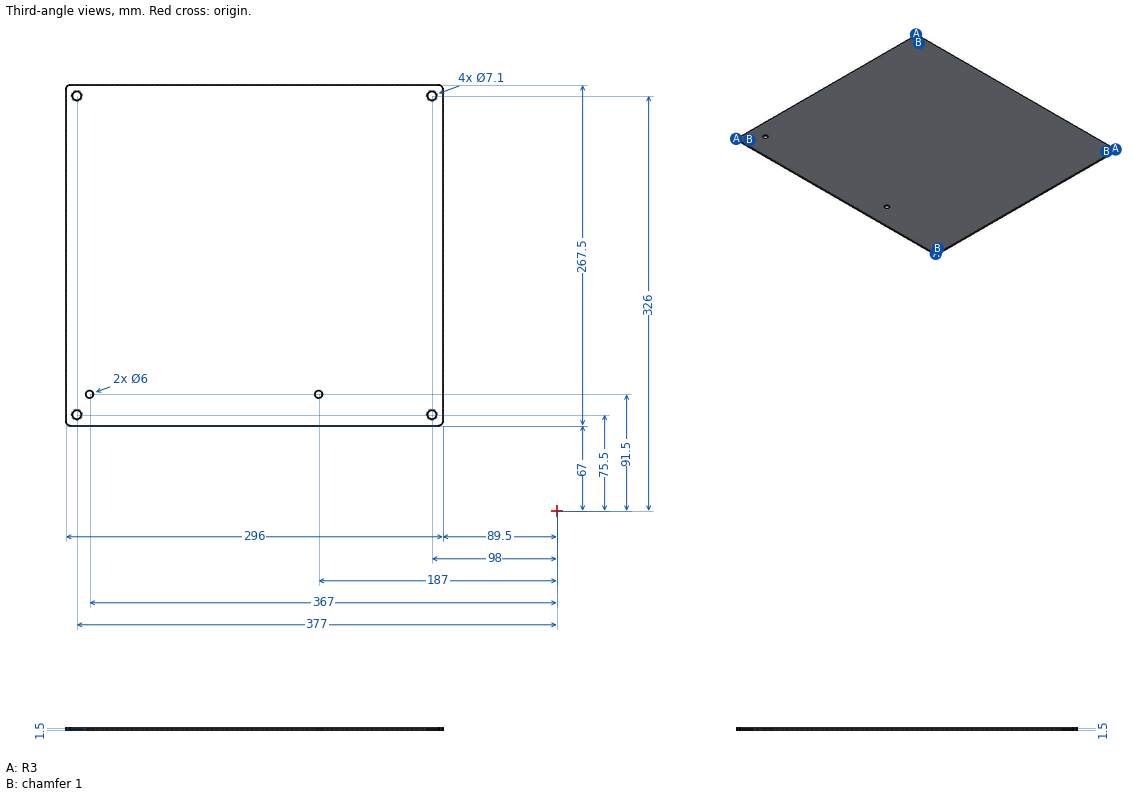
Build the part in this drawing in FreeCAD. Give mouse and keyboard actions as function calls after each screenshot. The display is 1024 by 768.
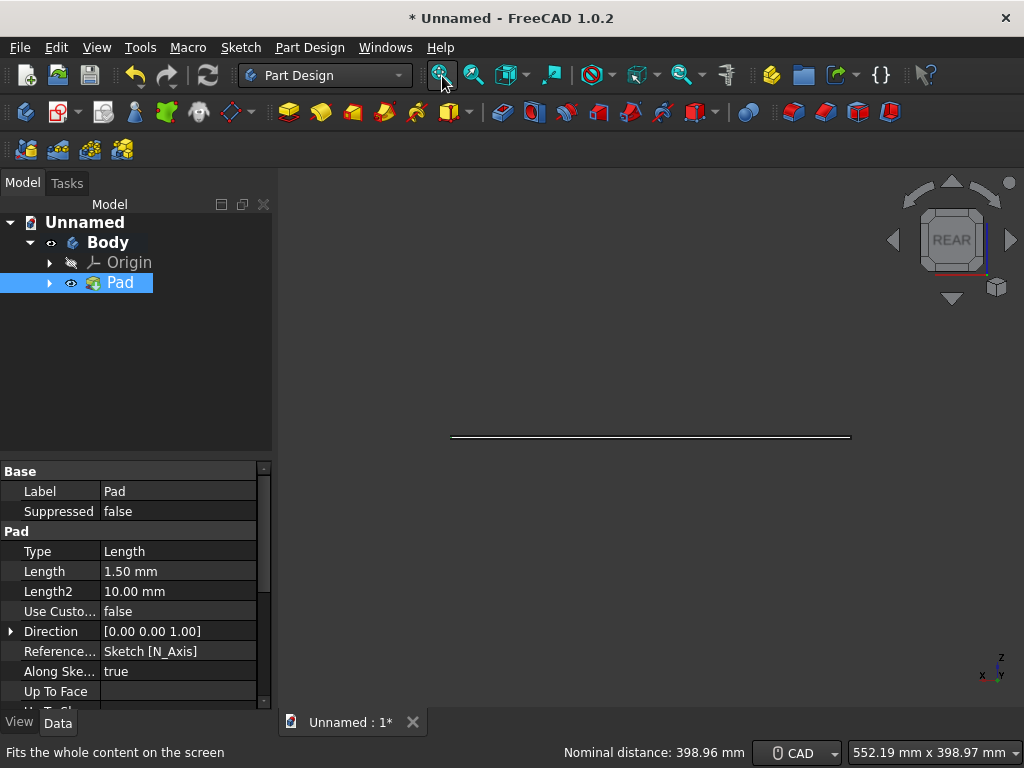
scroll(851, 436, up, 15)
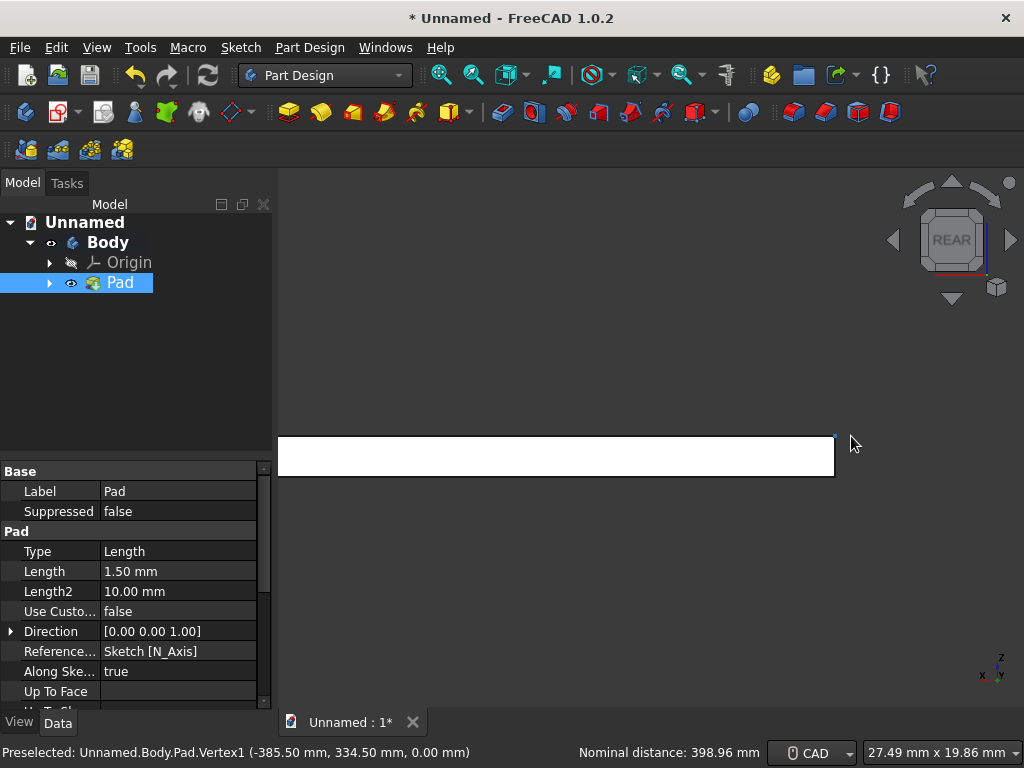
click(835, 456, ctrl)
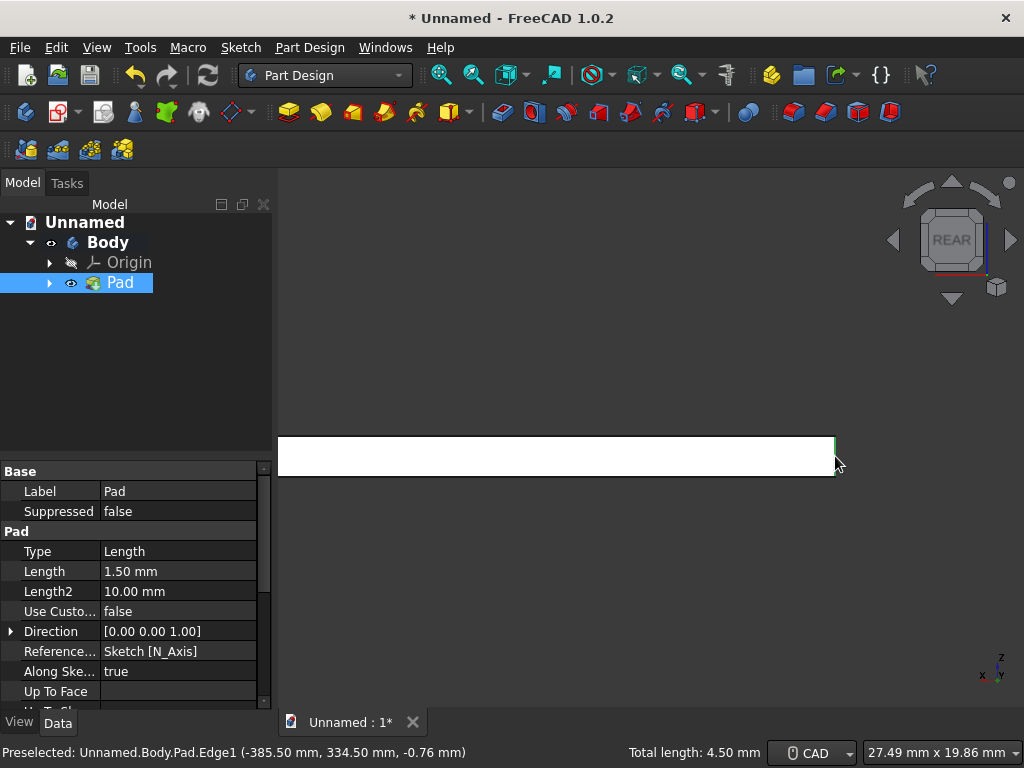
click(442, 76)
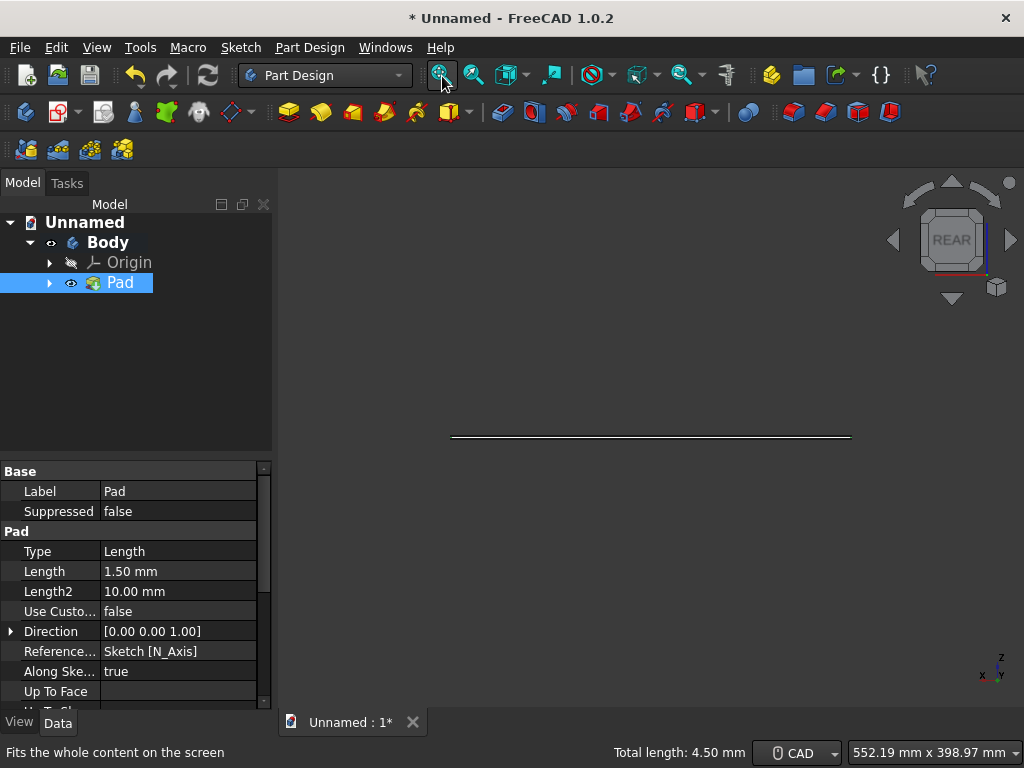
key(6)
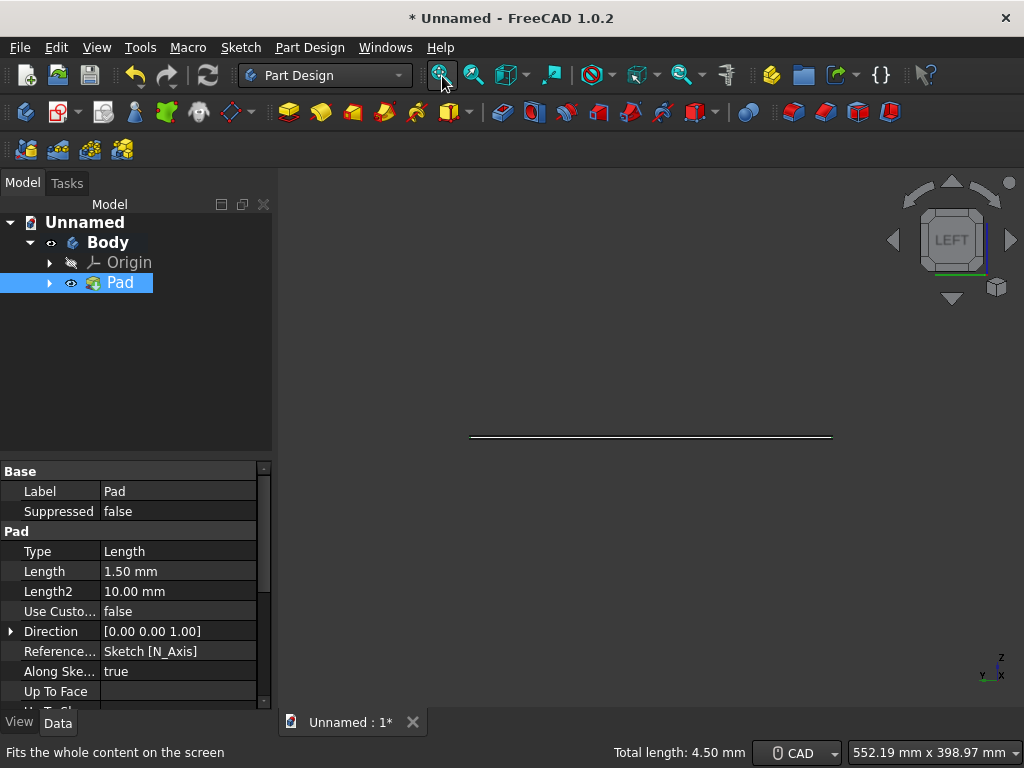
scroll(832, 436, up, 15)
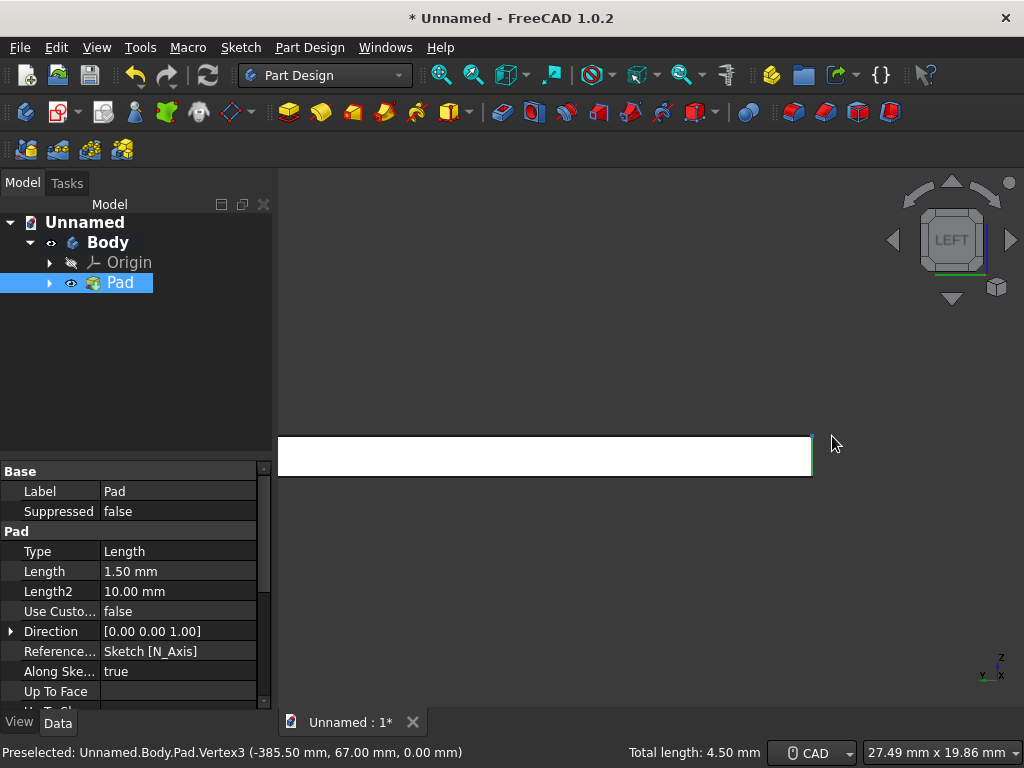
click(442, 76)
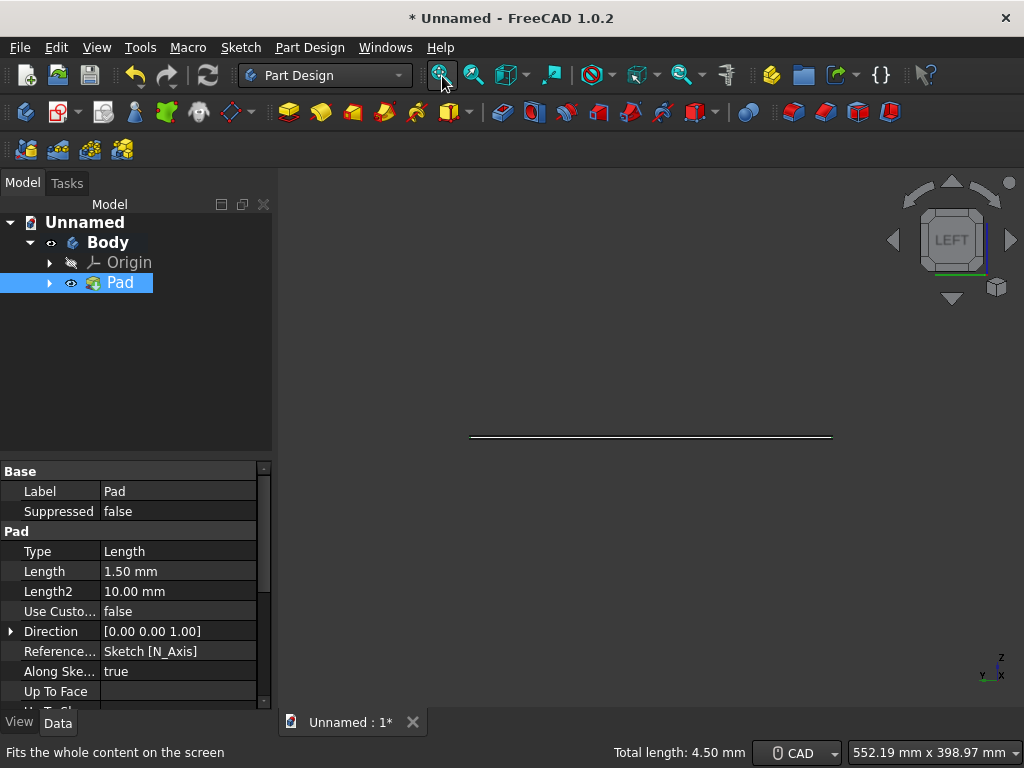
key(v)
key(3)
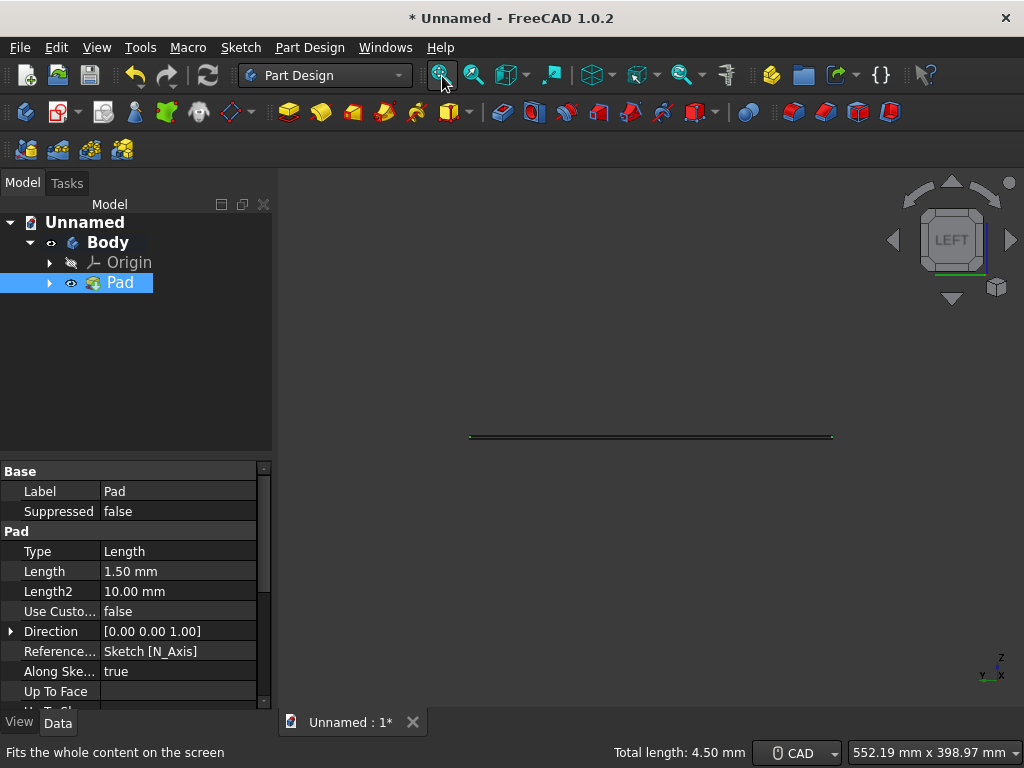
key(0)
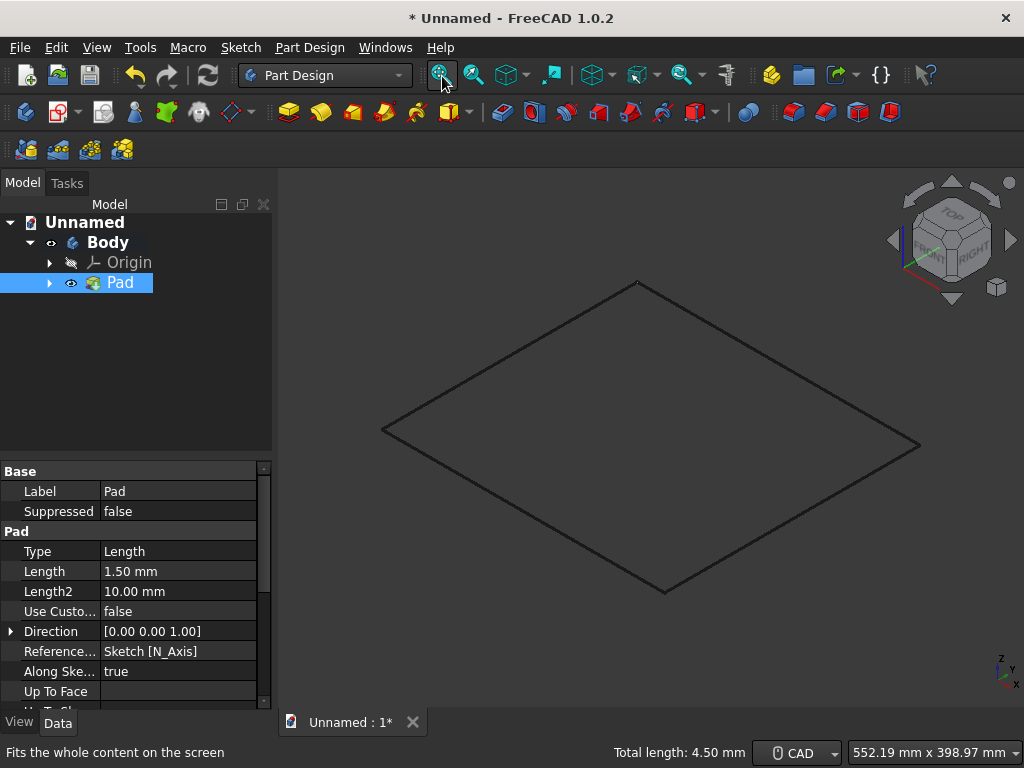
scroll(665, 592, up, 15)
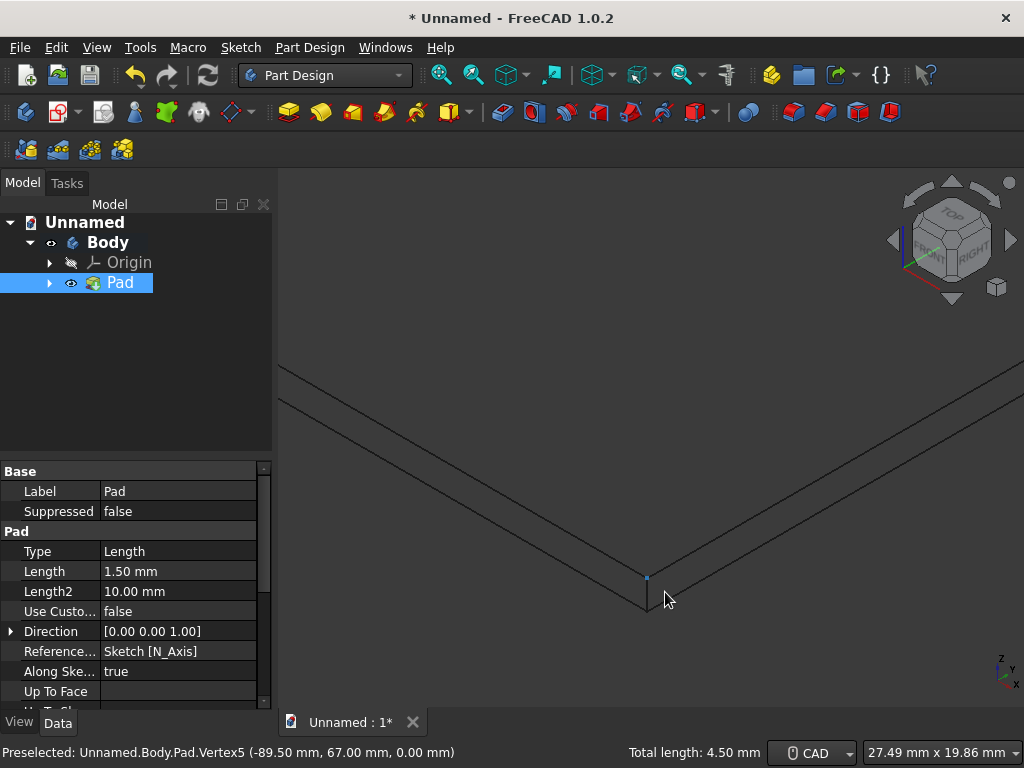
click(647, 594, ctrl)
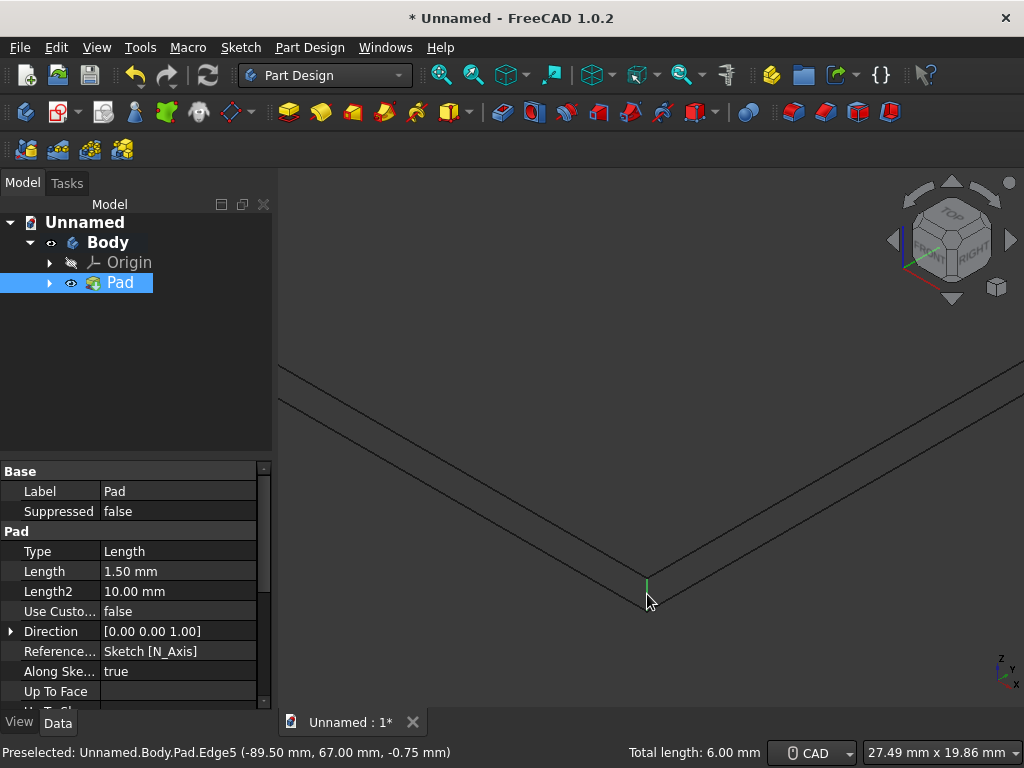
key(v)
key(1)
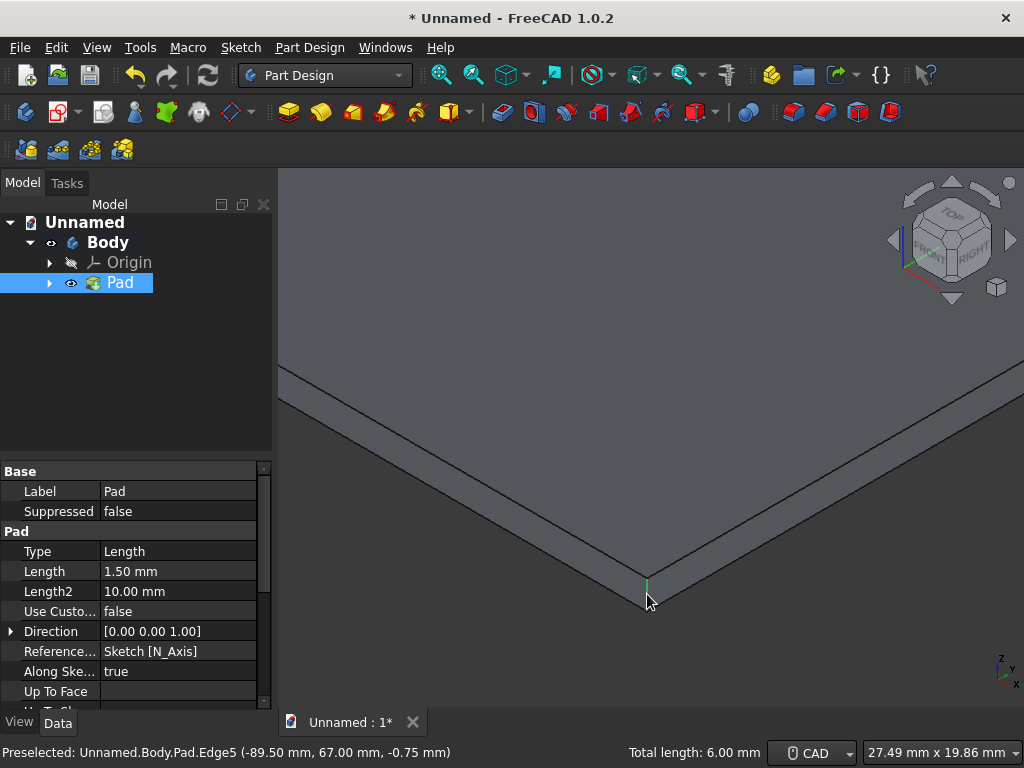
click(794, 112)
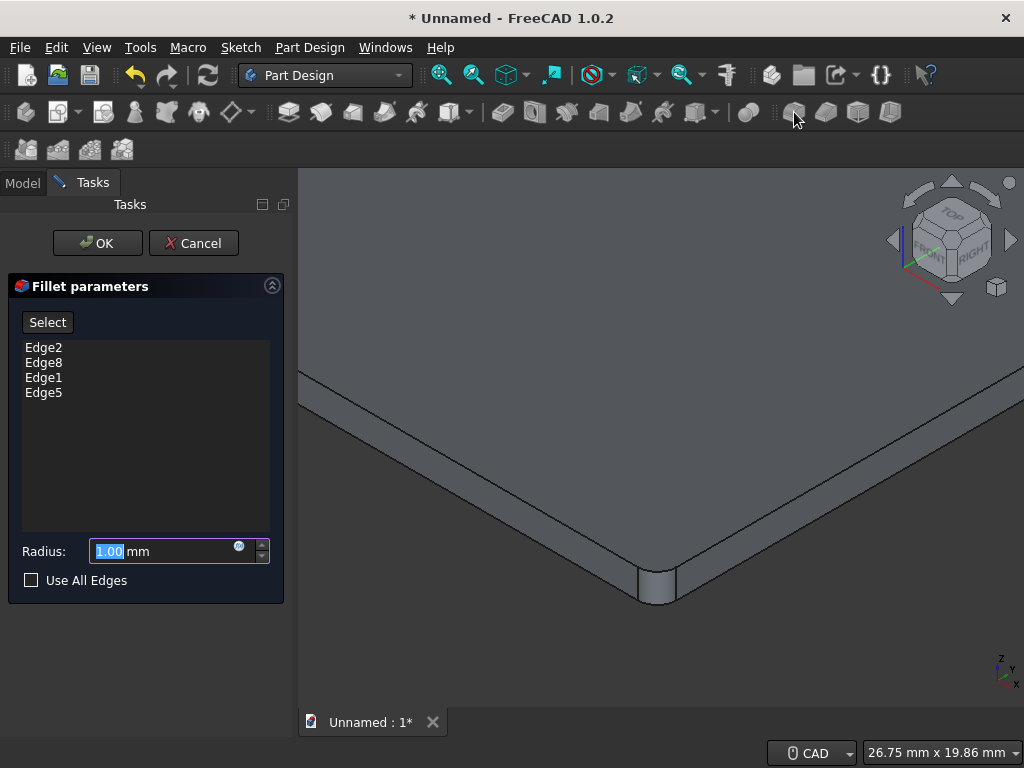
text(3)
key(Tab)